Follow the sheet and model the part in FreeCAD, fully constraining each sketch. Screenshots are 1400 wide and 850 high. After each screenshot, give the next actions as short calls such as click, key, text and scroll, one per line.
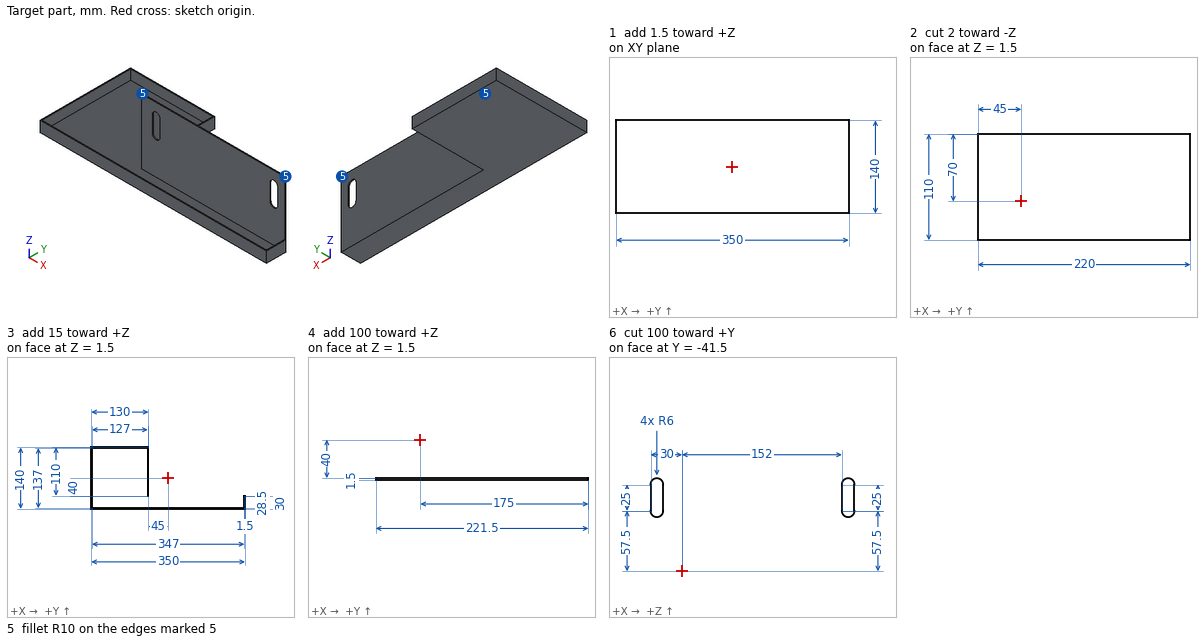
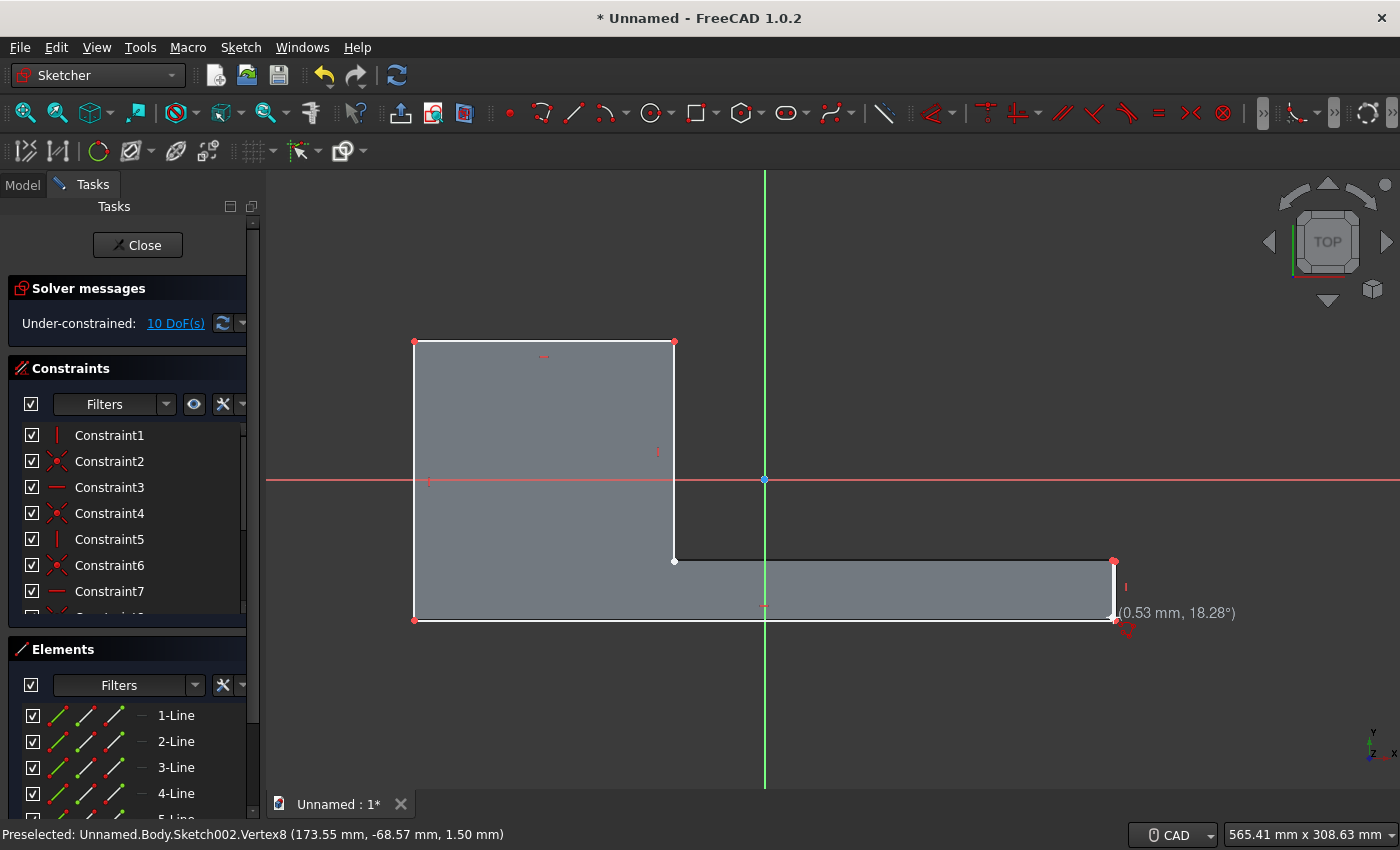
scroll(417, 617, up, 9)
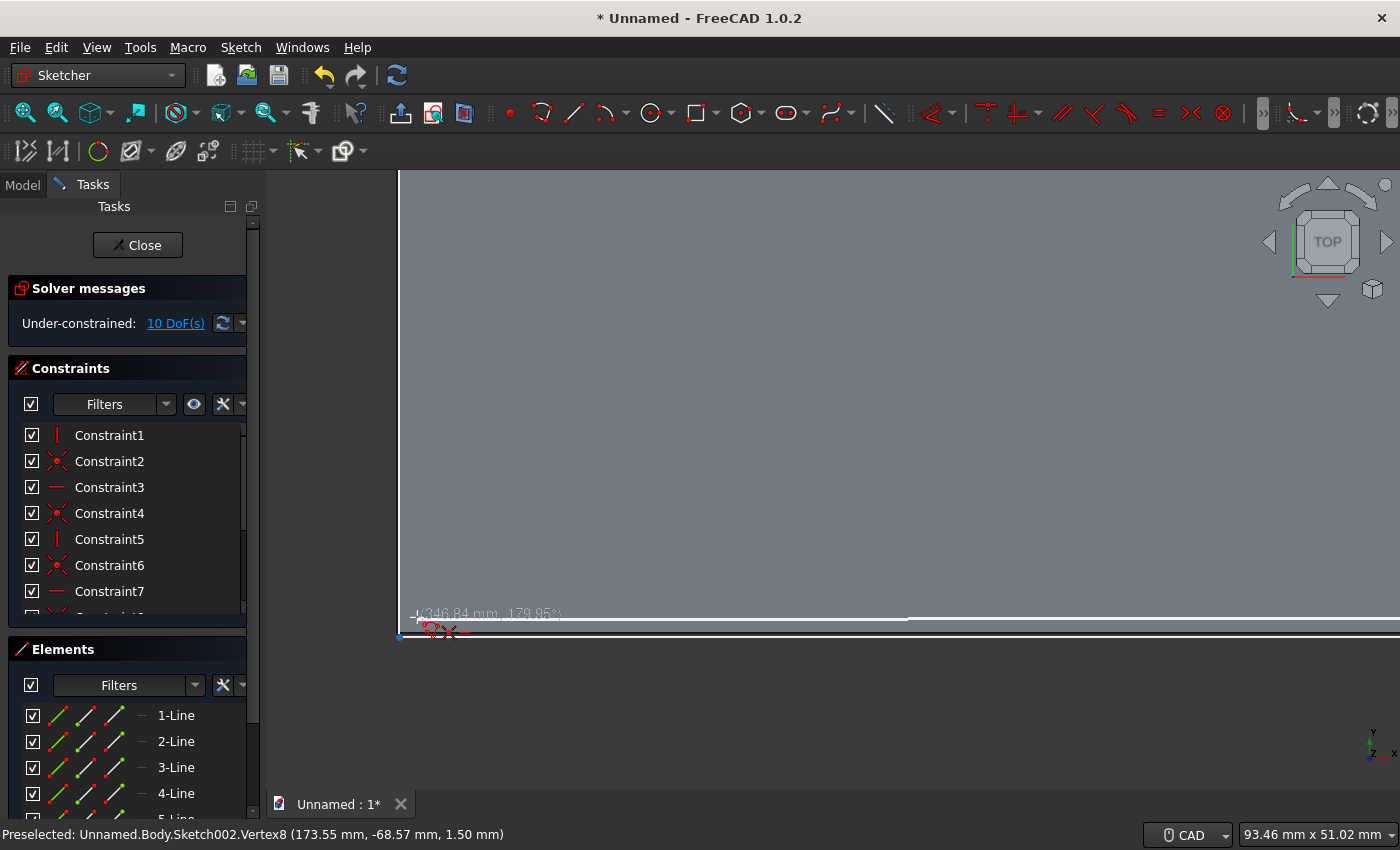
click(415, 615)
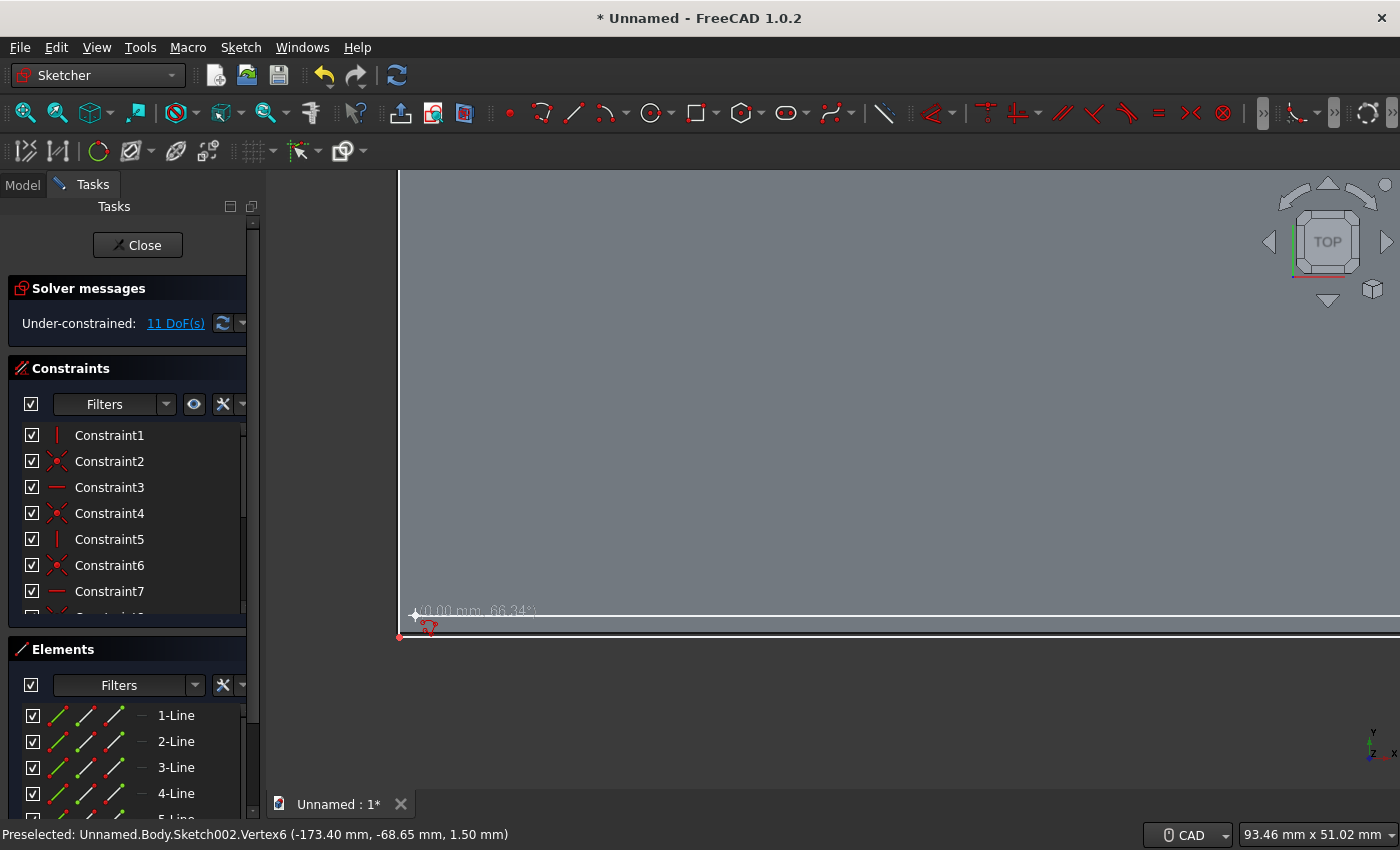
scroll(417, 617, down, 9)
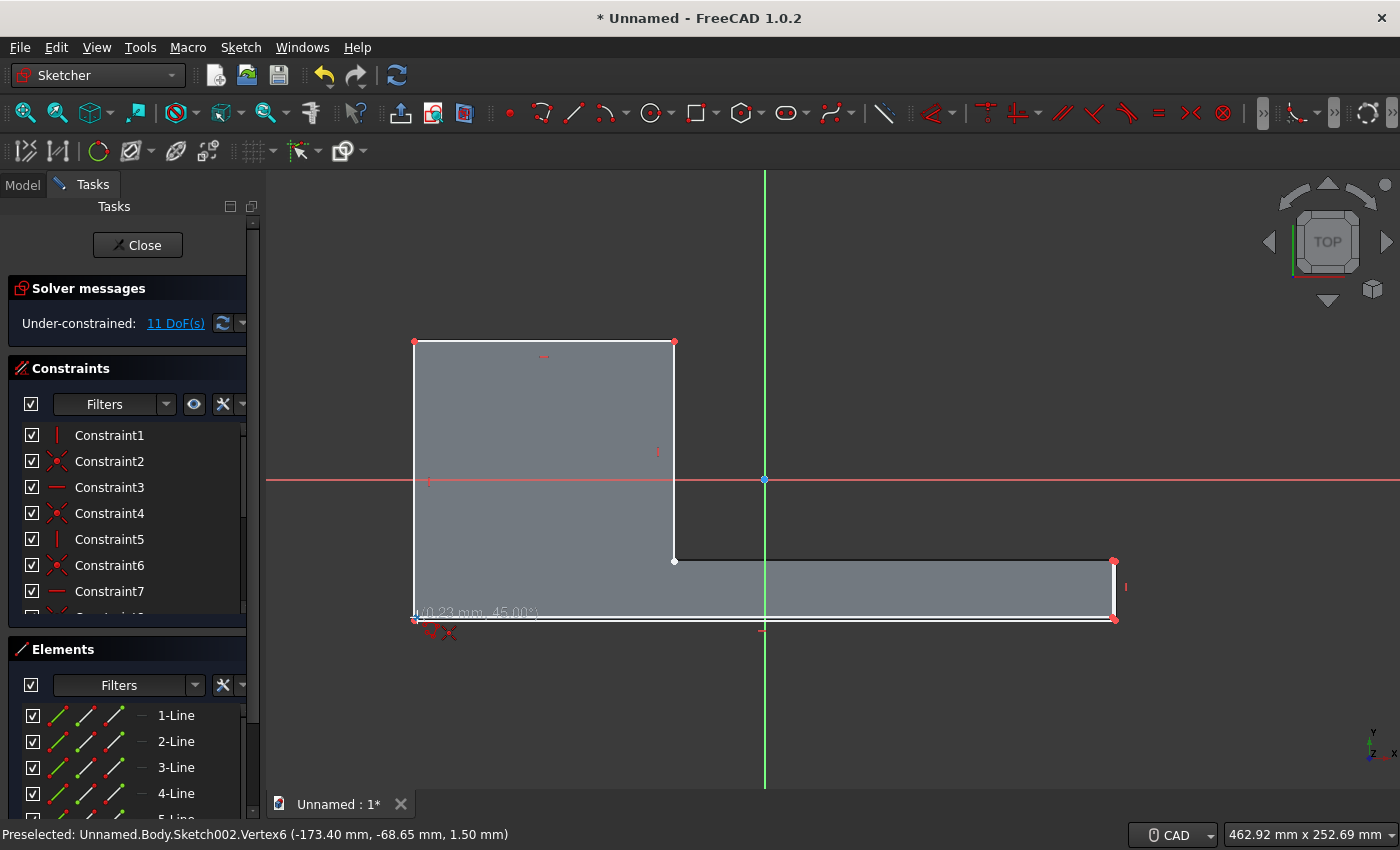
scroll(417, 343, up, 9)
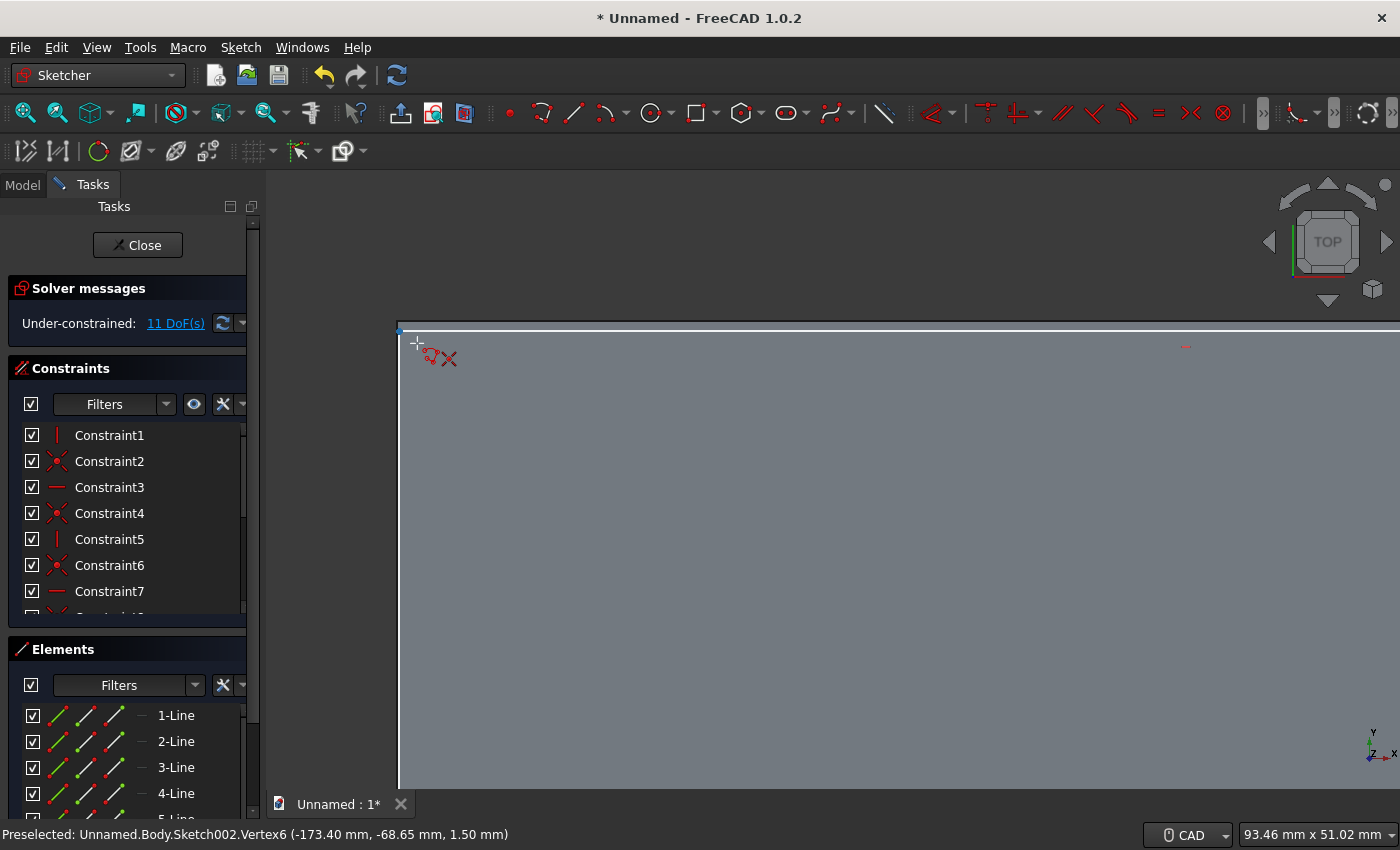
click(415, 339)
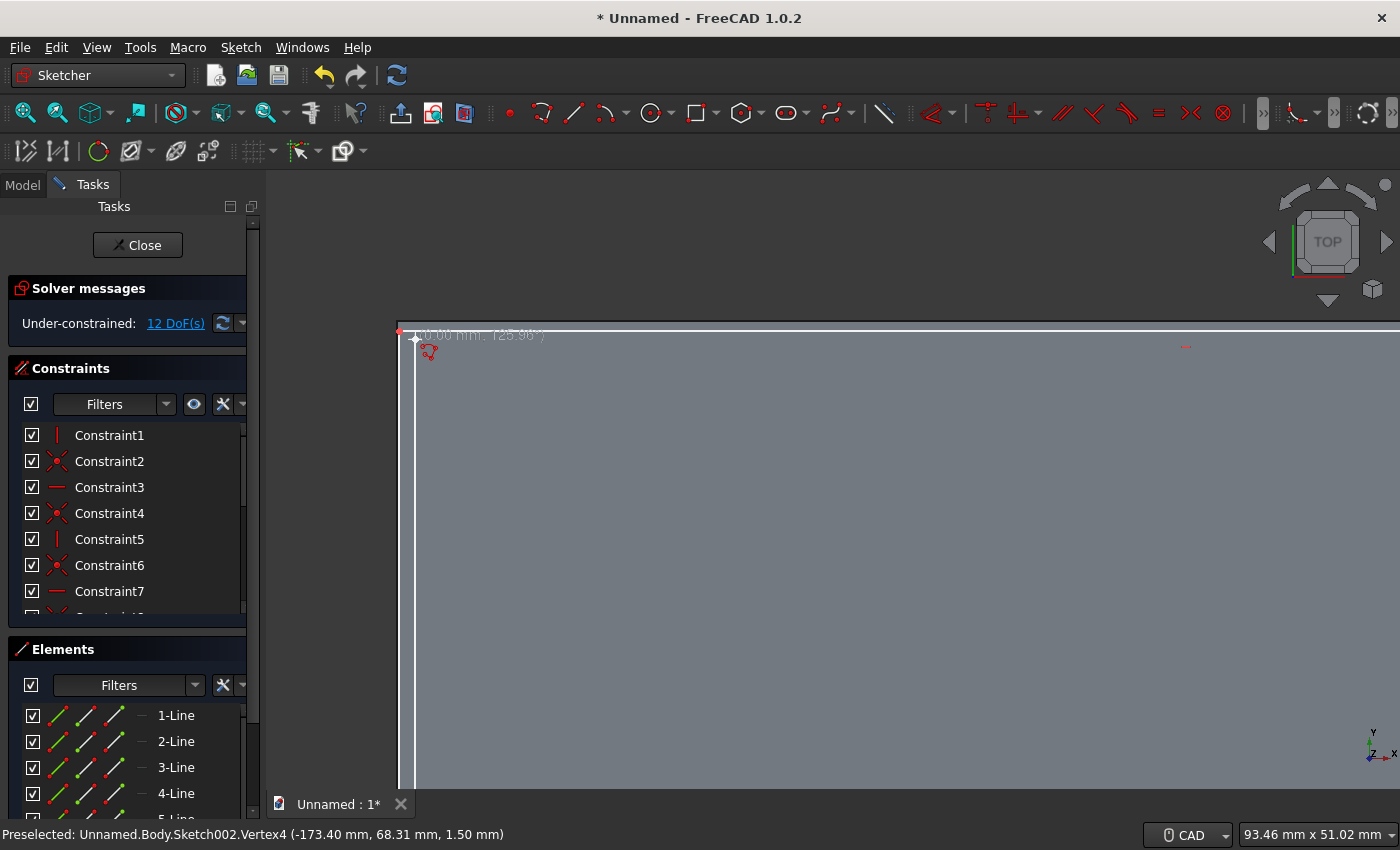
scroll(417, 343, down, 9)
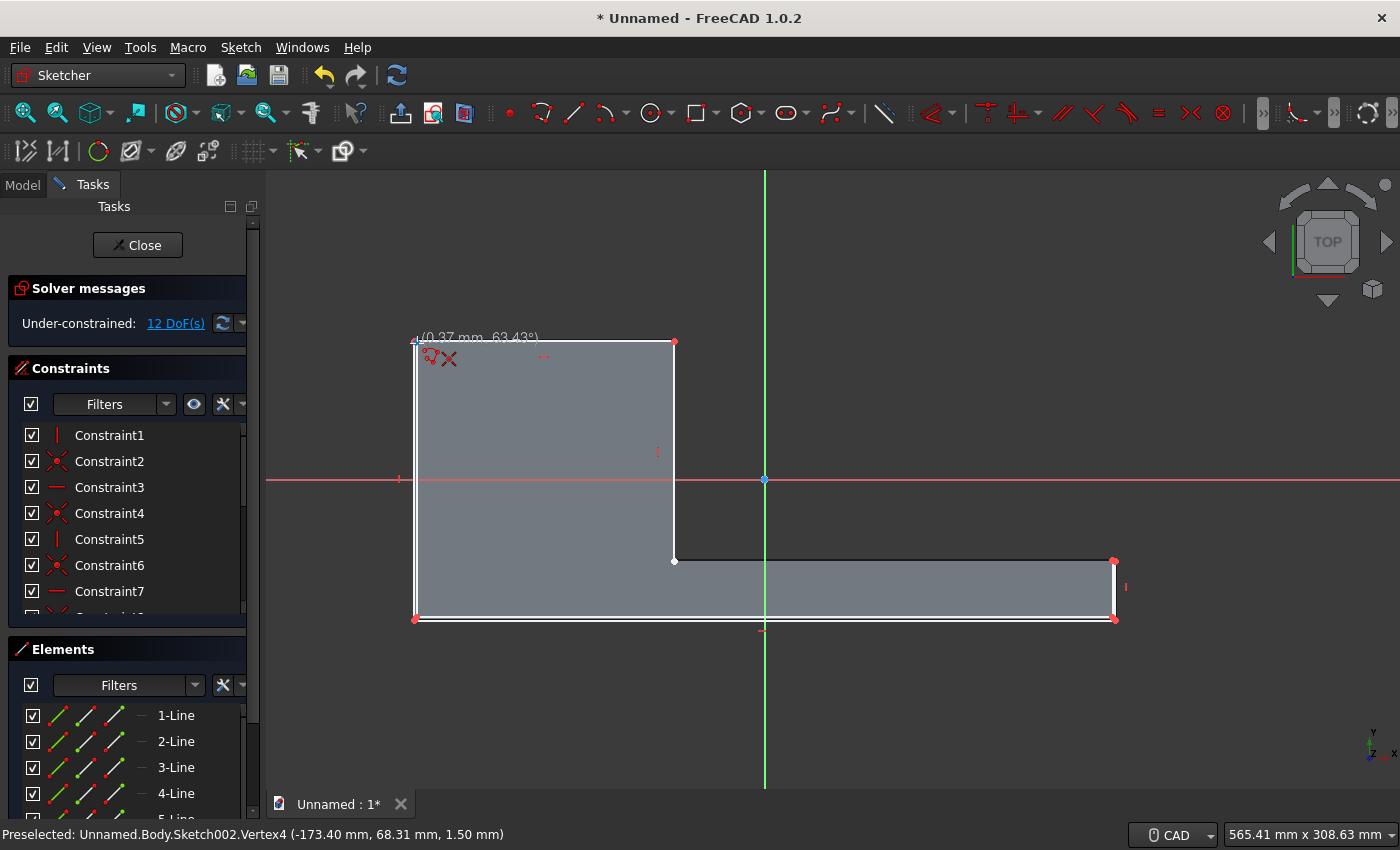
scroll(671, 343, up, 9)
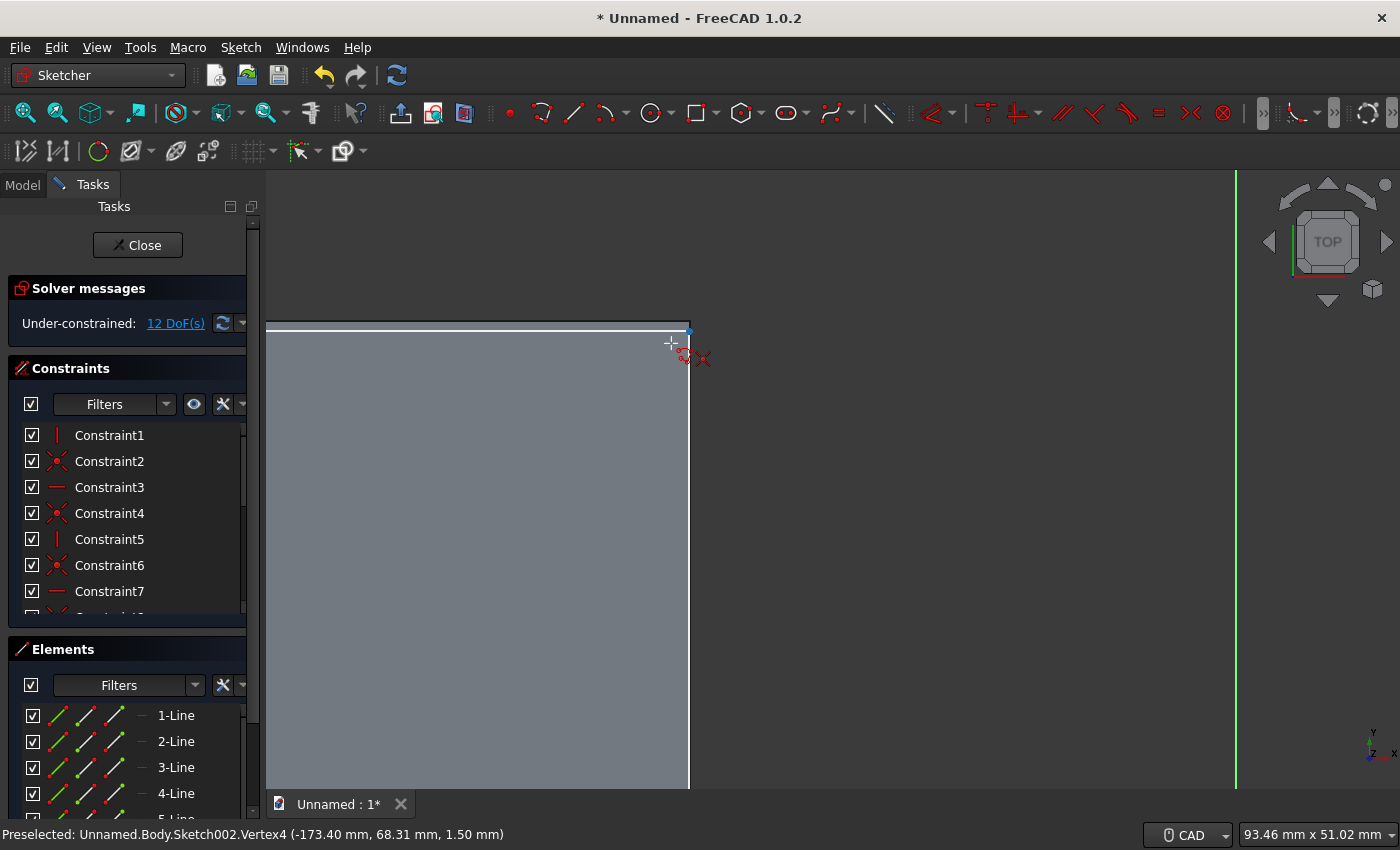
click(672, 339)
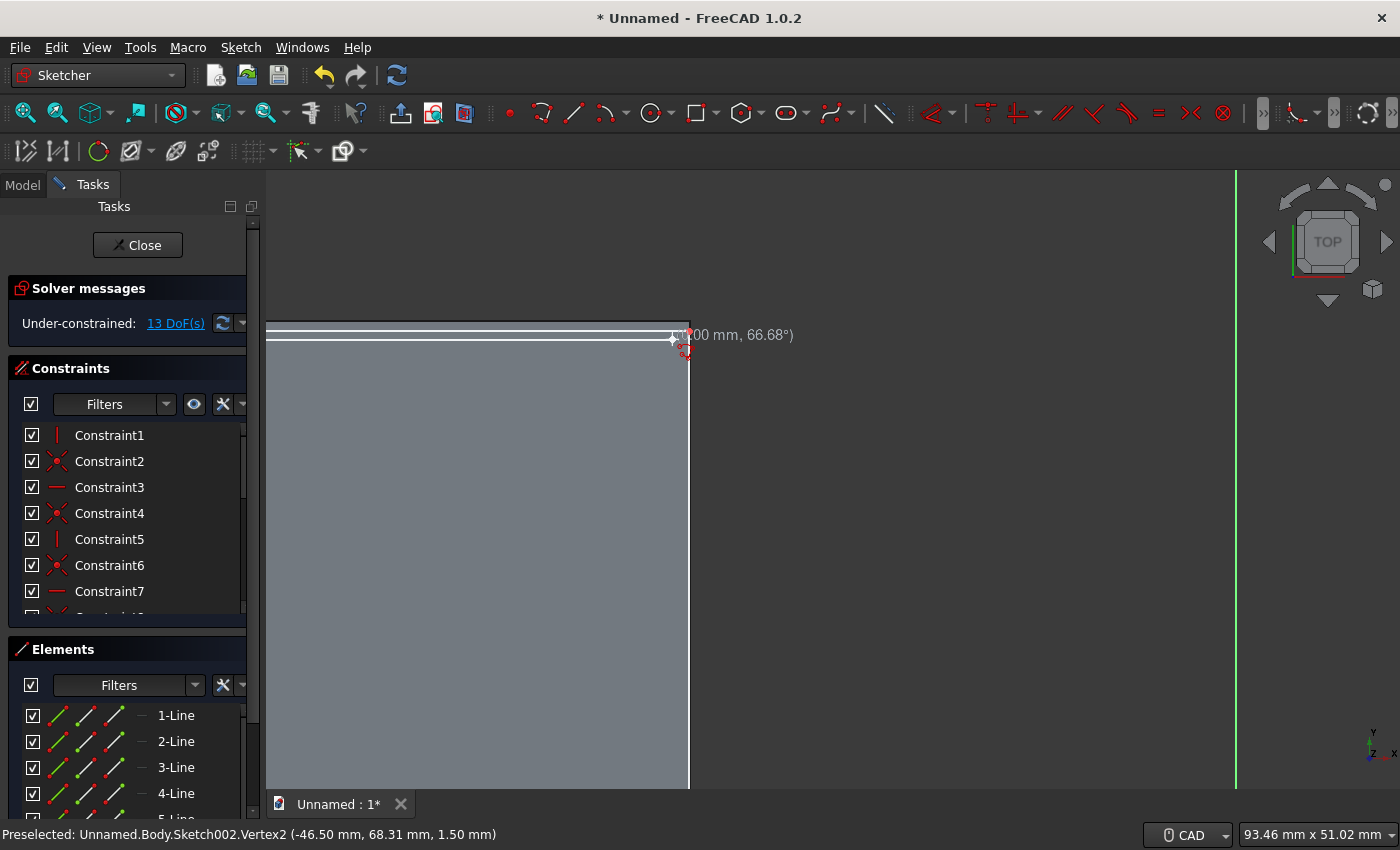
scroll(671, 343, down, 9)